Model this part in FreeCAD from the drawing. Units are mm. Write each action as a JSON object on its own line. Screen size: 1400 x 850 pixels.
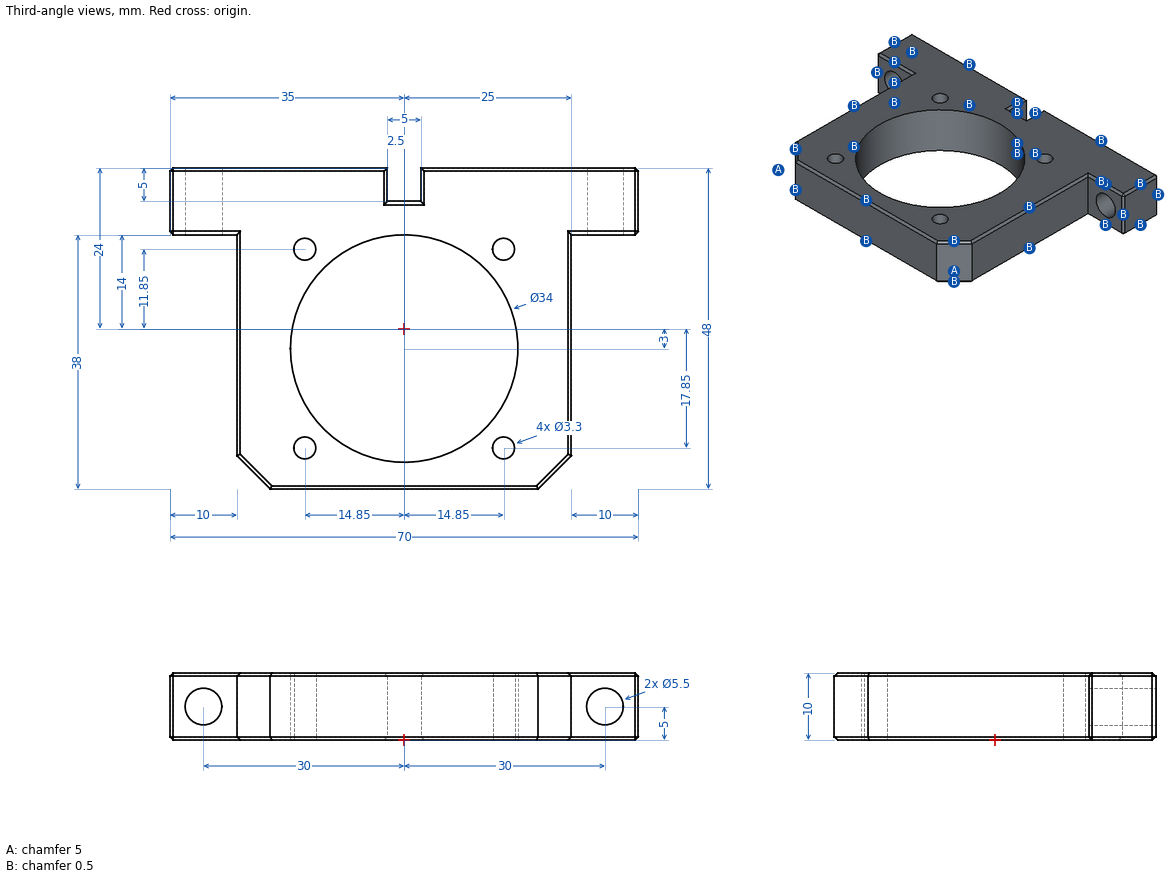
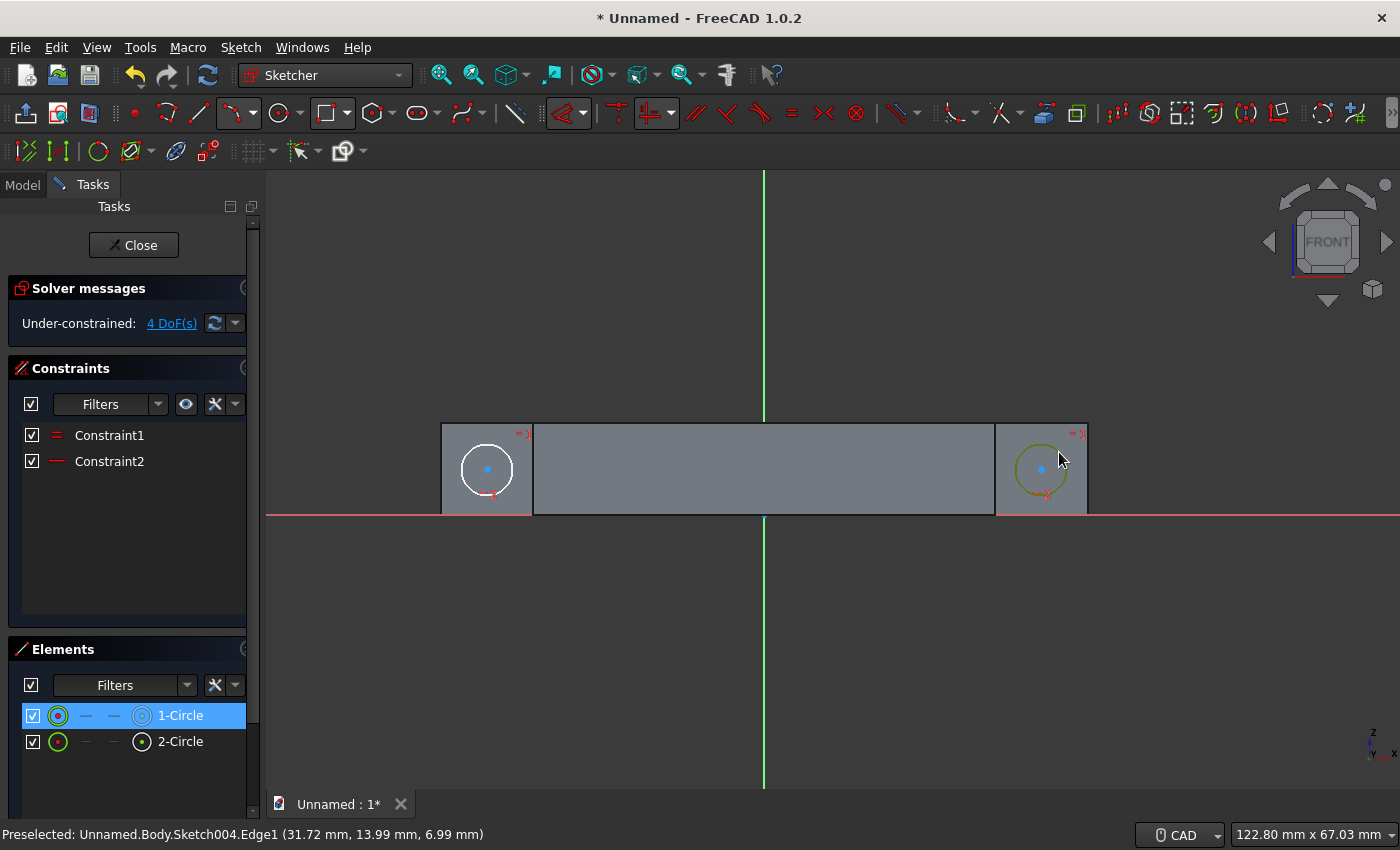
{"action": "left_click", "coordinate": [586, 114]}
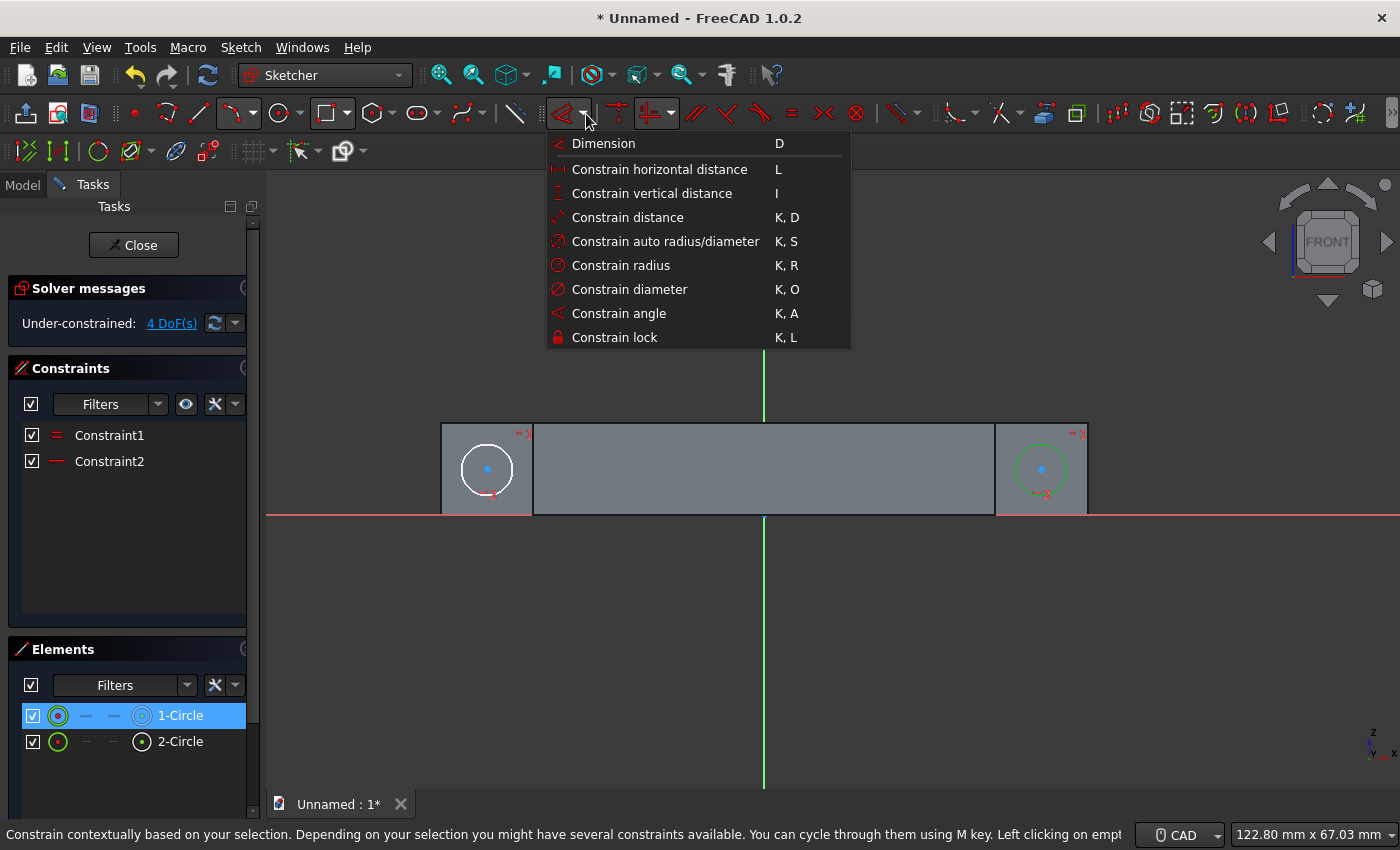
{"action": "left_click", "coordinate": [699, 289]}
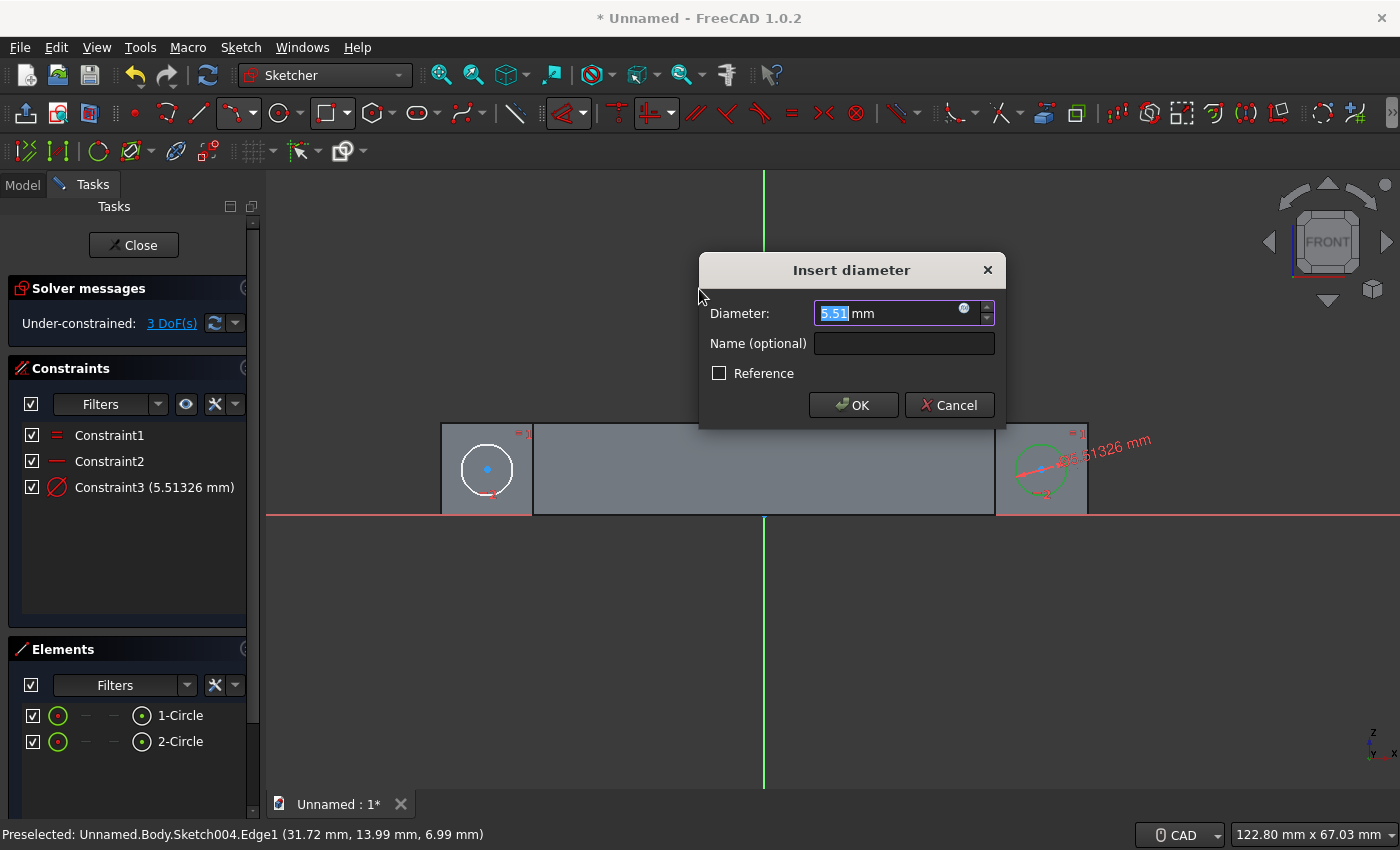
{"action": "type", "text": "5.5"}
{"action": "key", "text": "Return"}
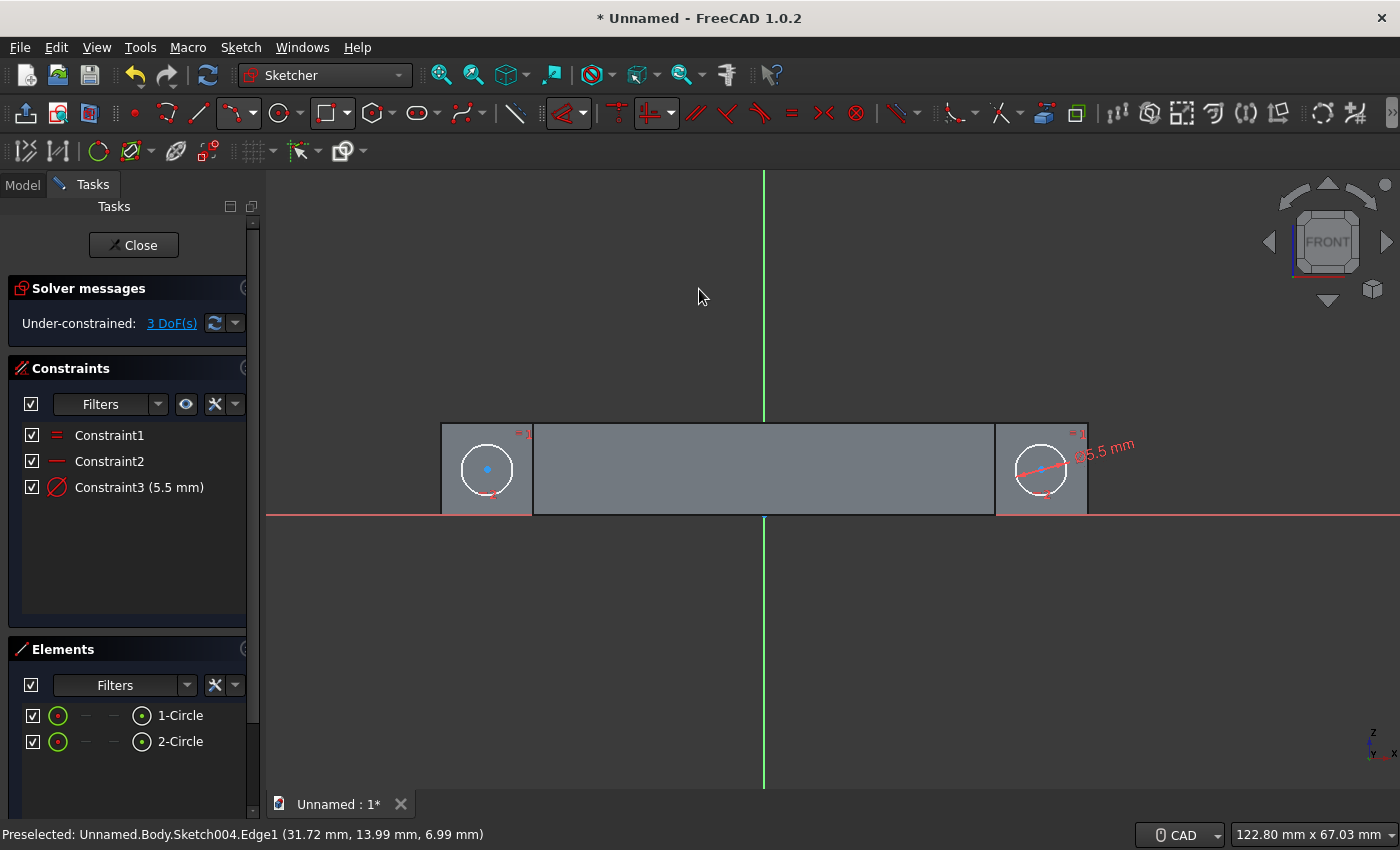
{"action": "left_click", "coordinate": [1041, 470]}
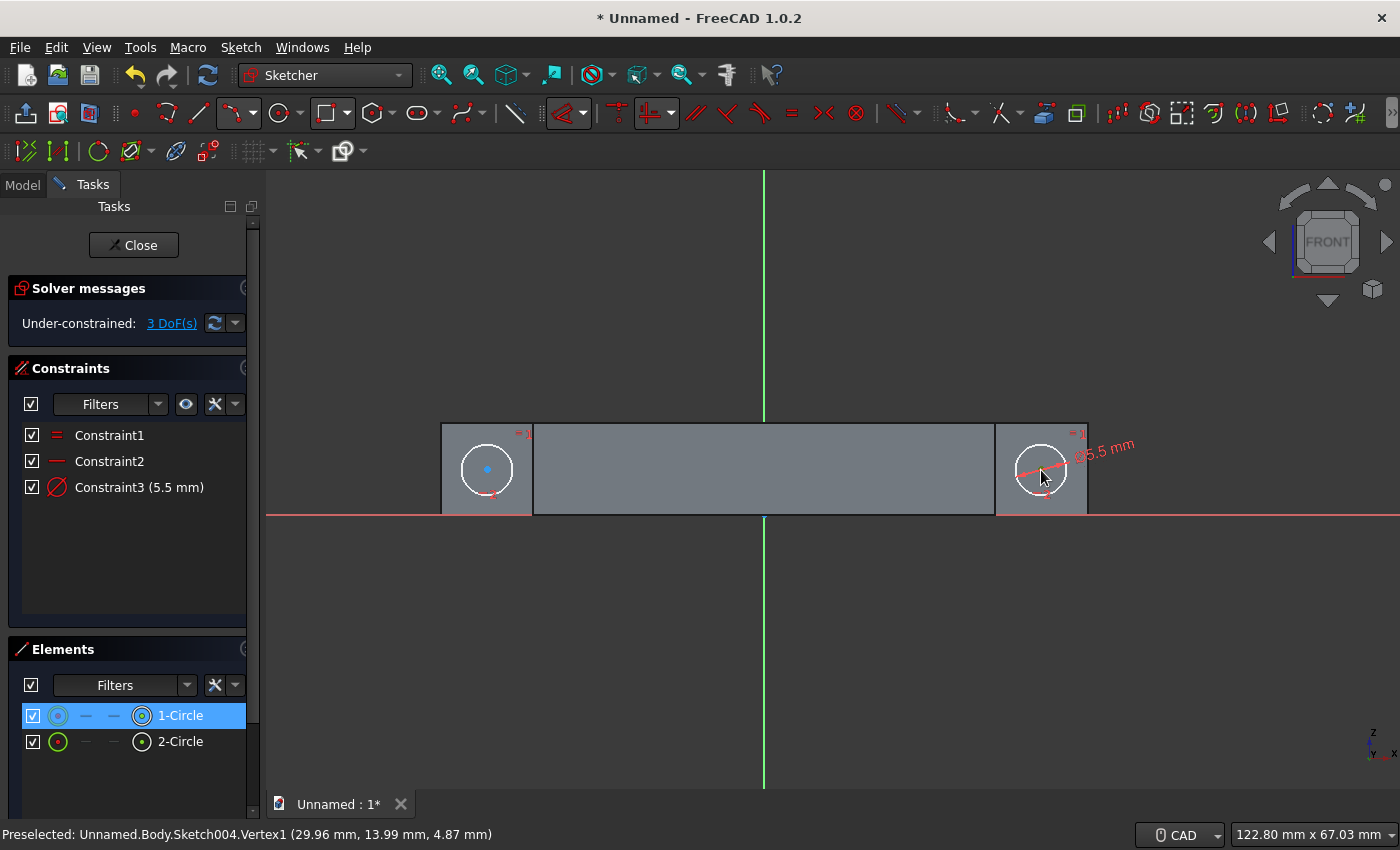
{"action": "key", "text": "i"}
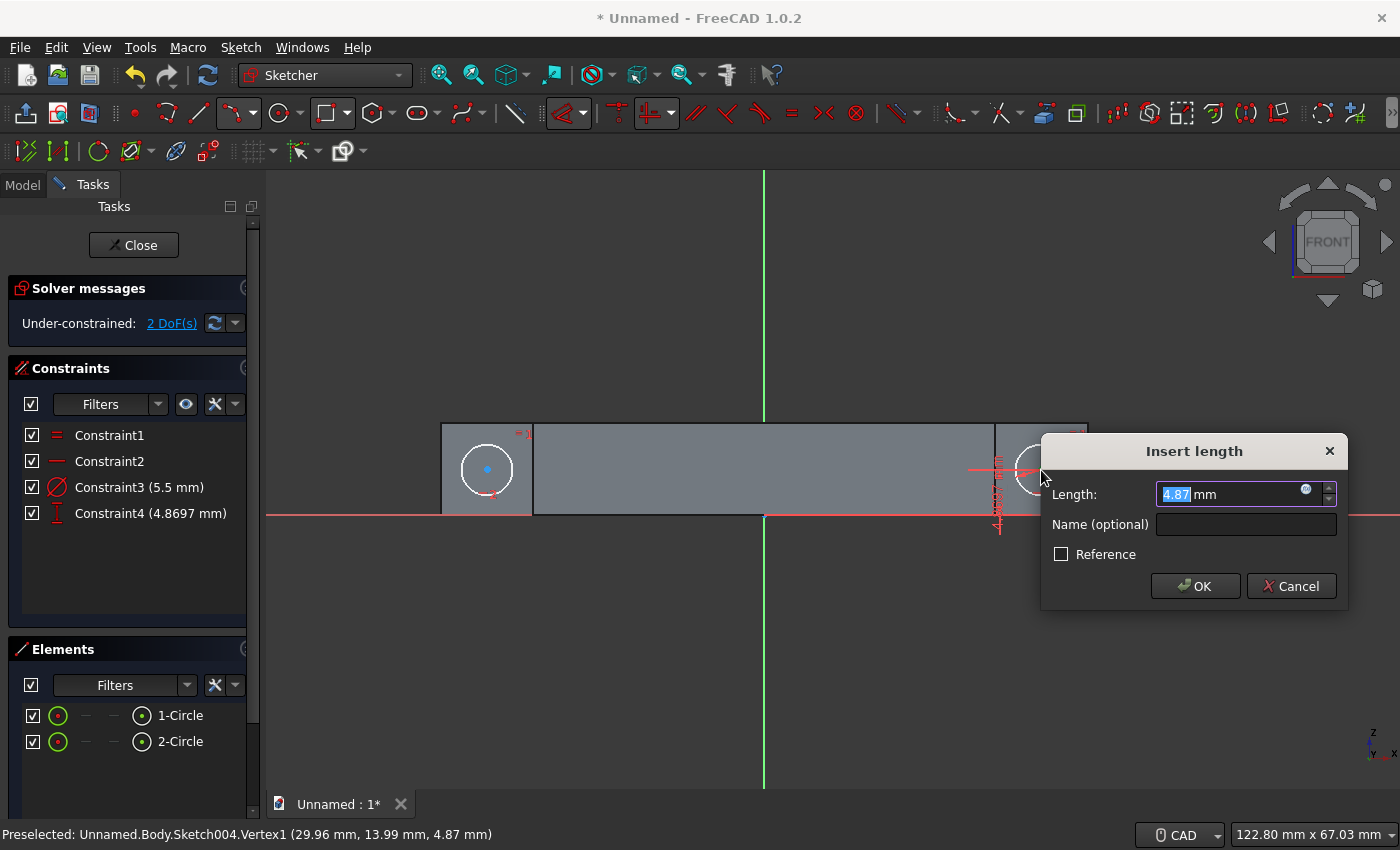
{"action": "type", "text": "5"}
{"action": "key", "text": "Return"}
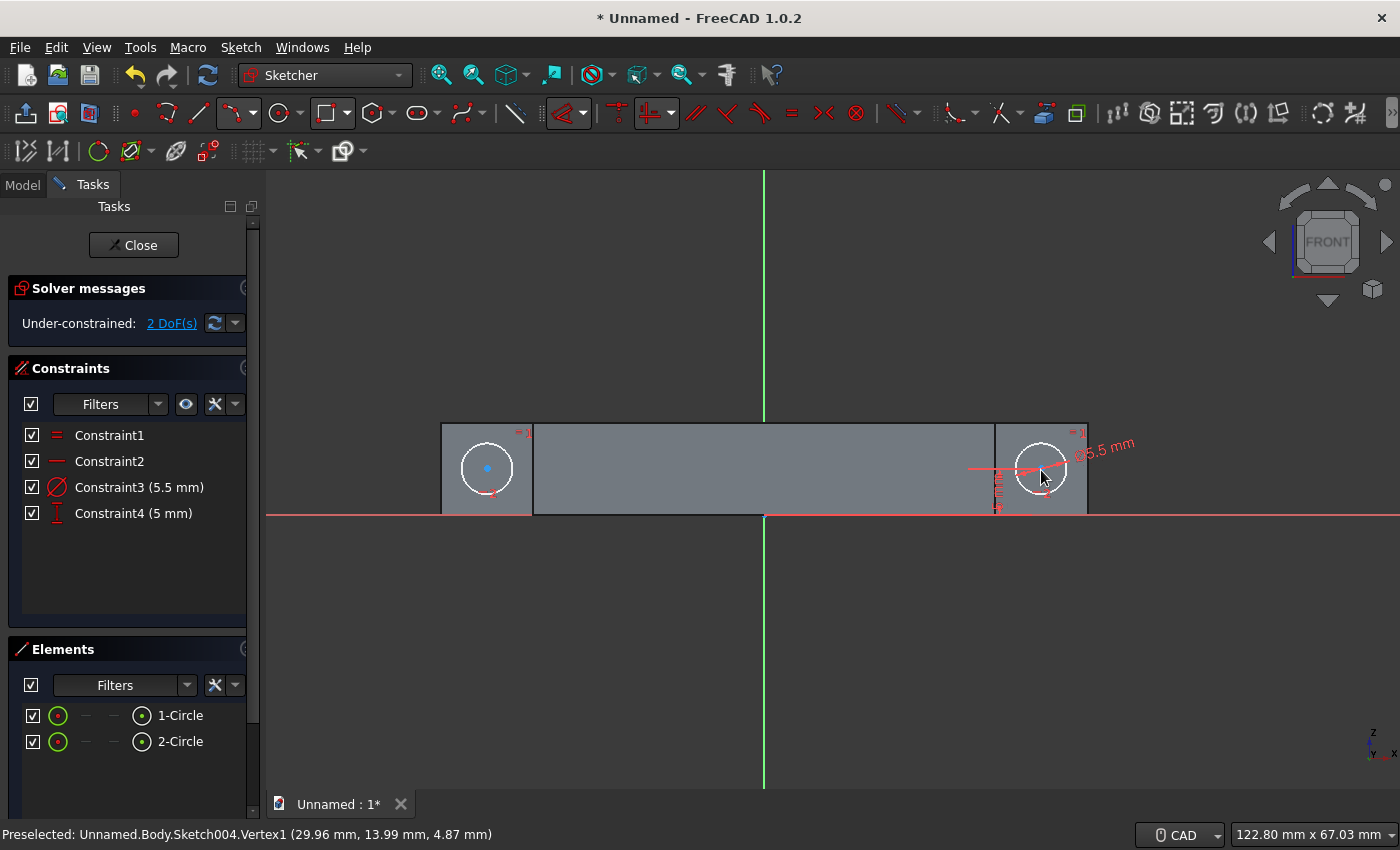
{"action": "left_click", "coordinate": [1041, 469]}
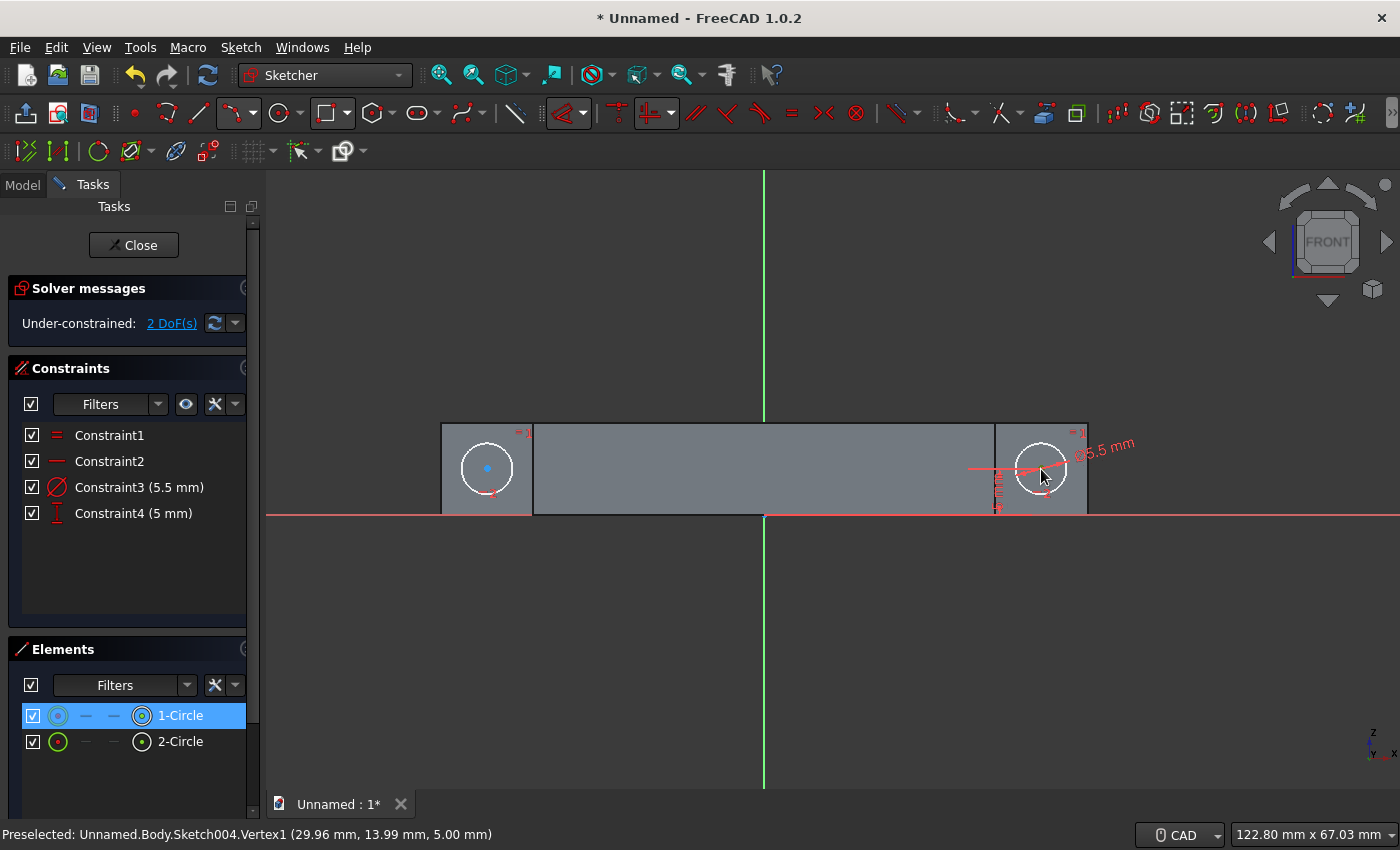
{"action": "left_click", "coordinate": [586, 114]}